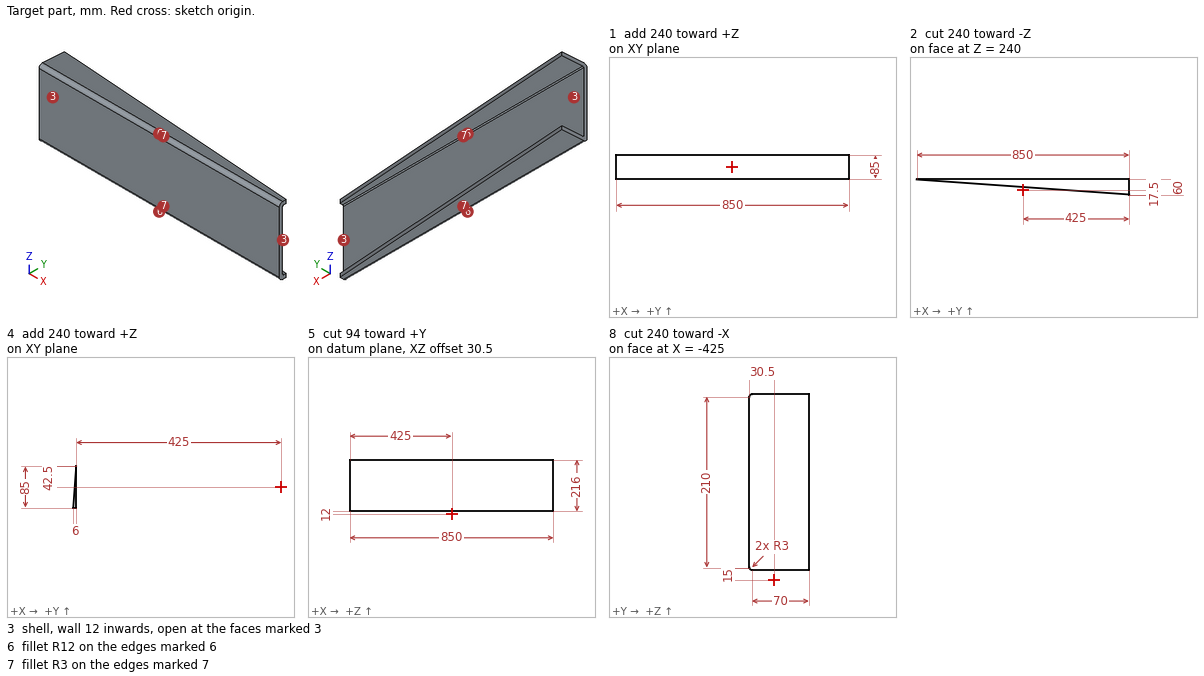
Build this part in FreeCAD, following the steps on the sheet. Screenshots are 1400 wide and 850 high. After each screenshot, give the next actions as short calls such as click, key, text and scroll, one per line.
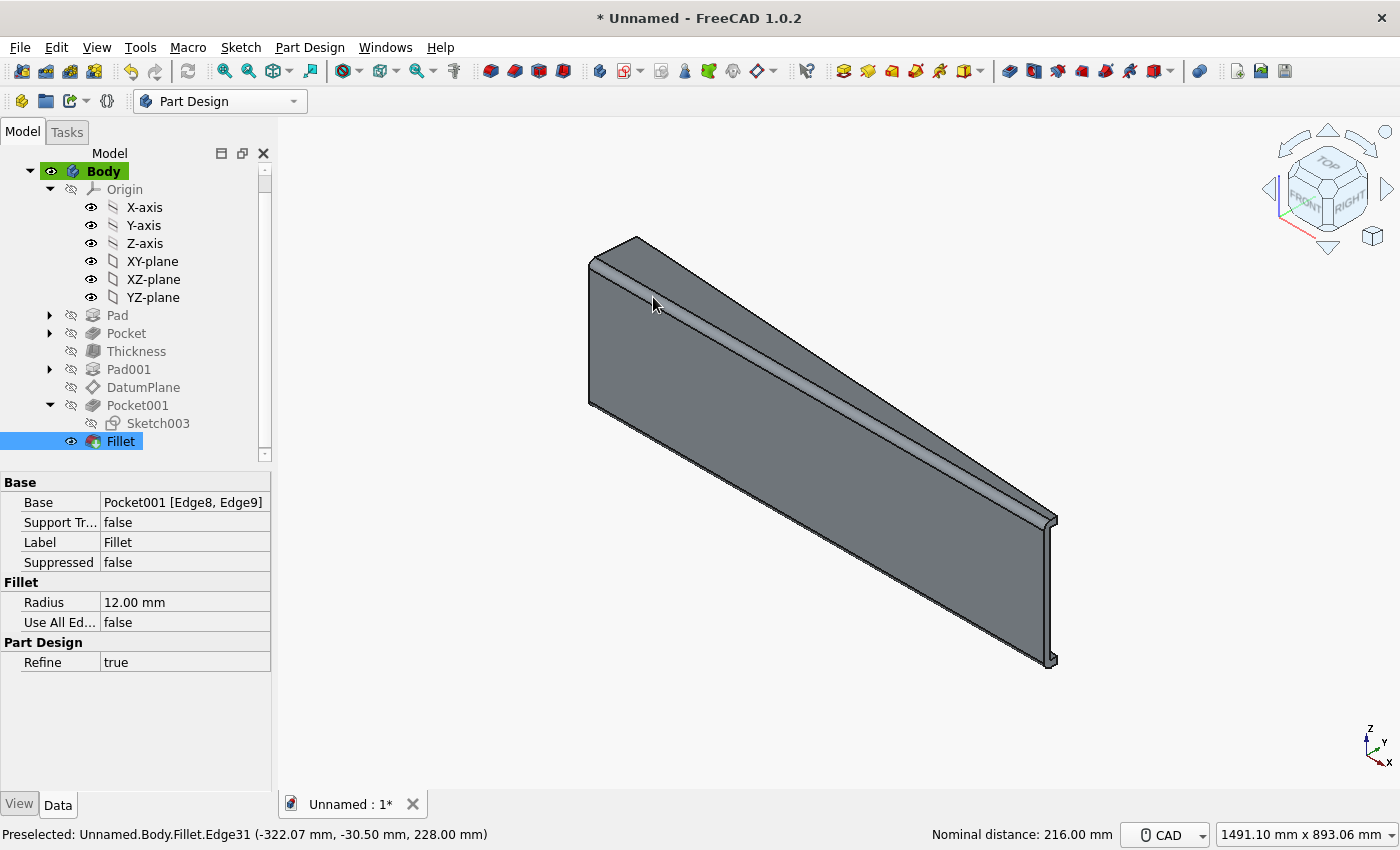
click(492, 72)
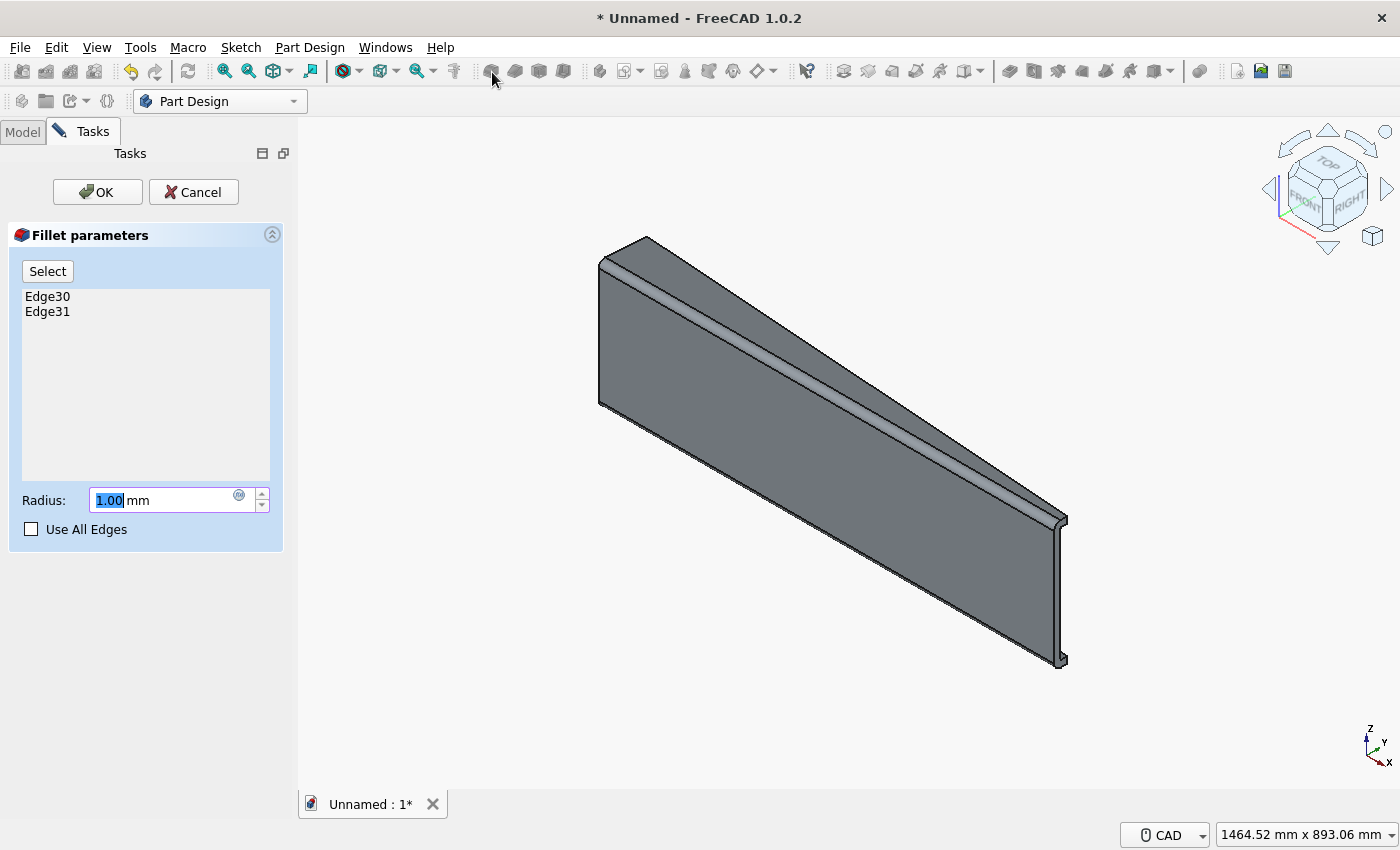
text(3)
key(Tab)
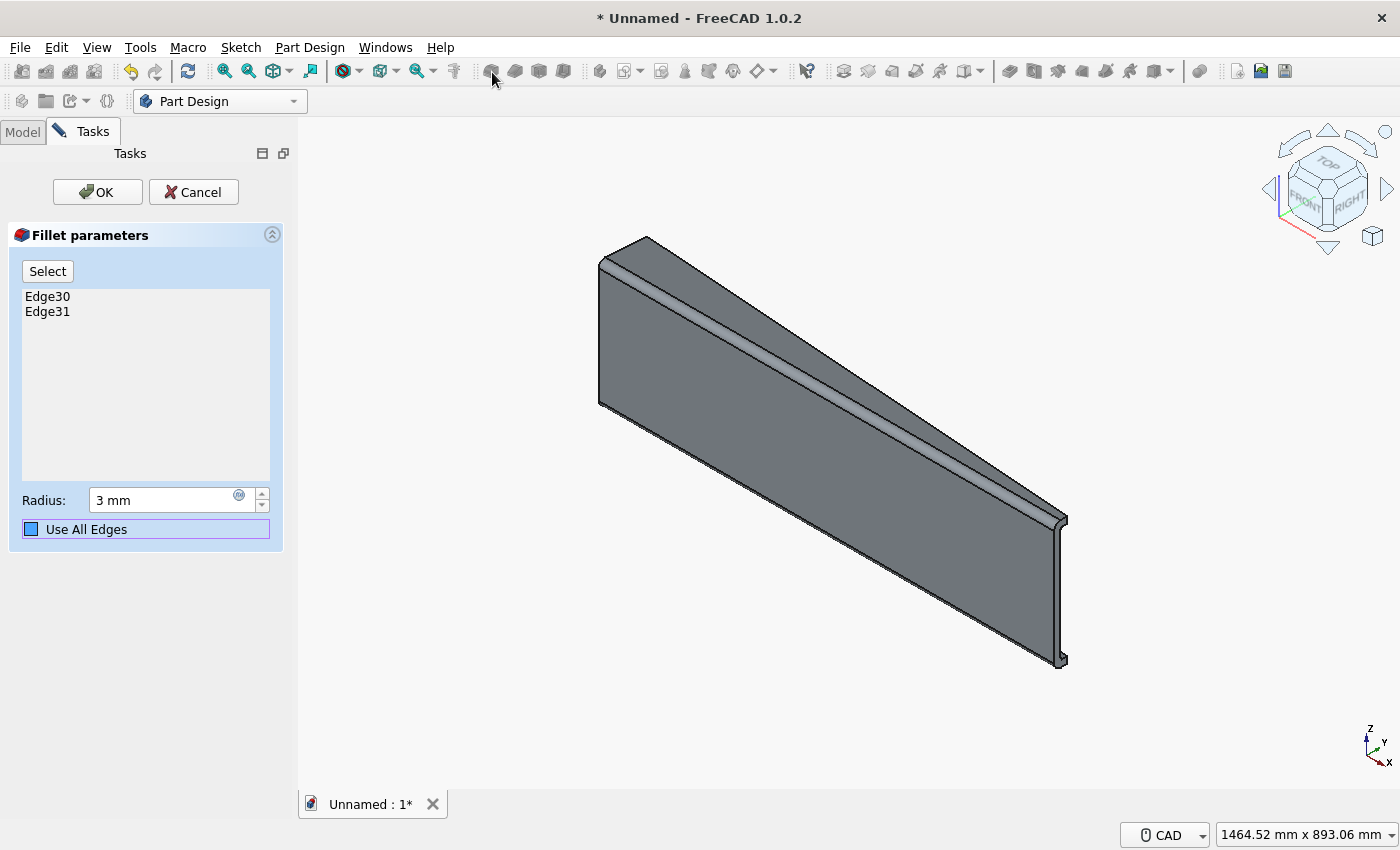
click(98, 192)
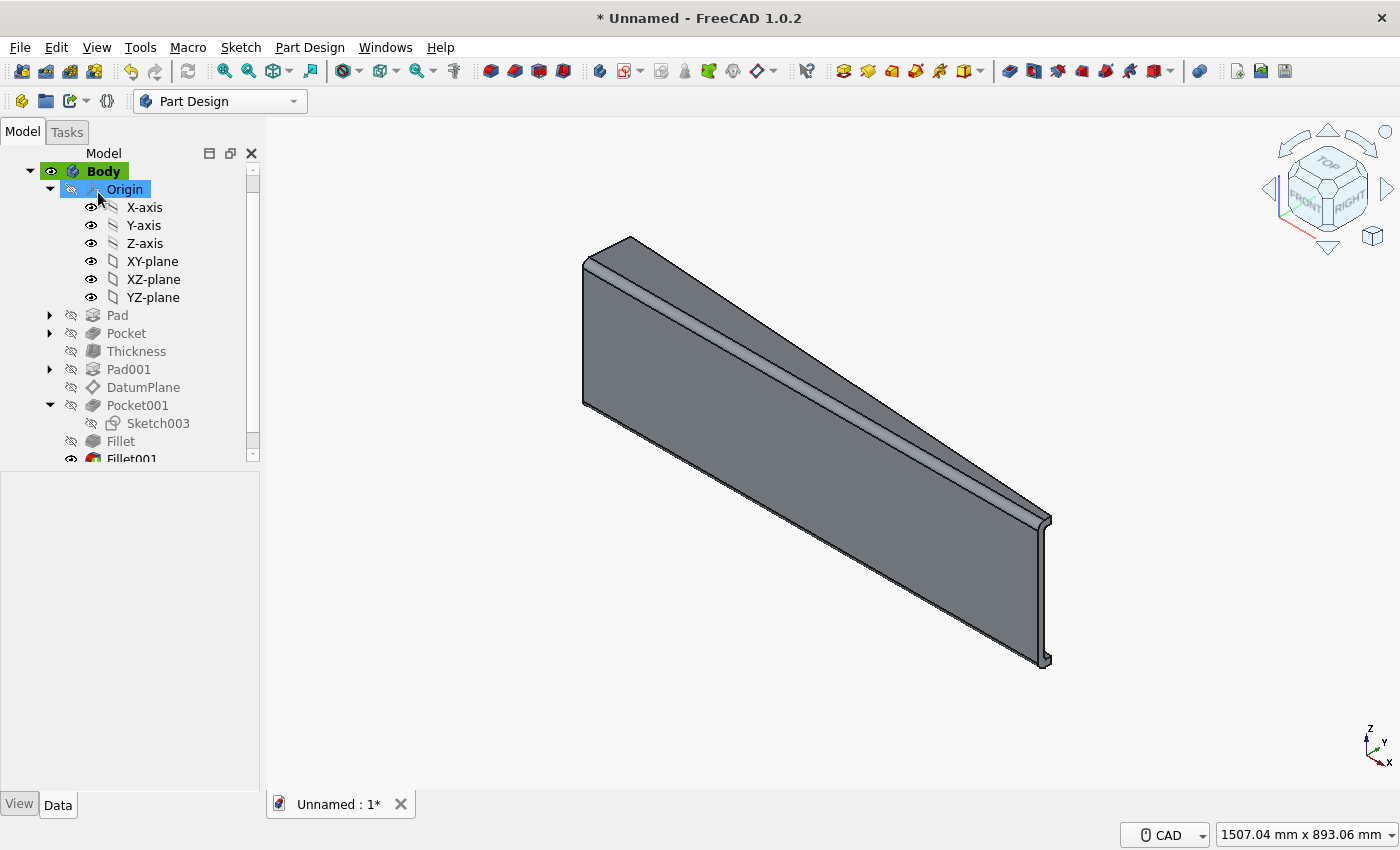
key(3)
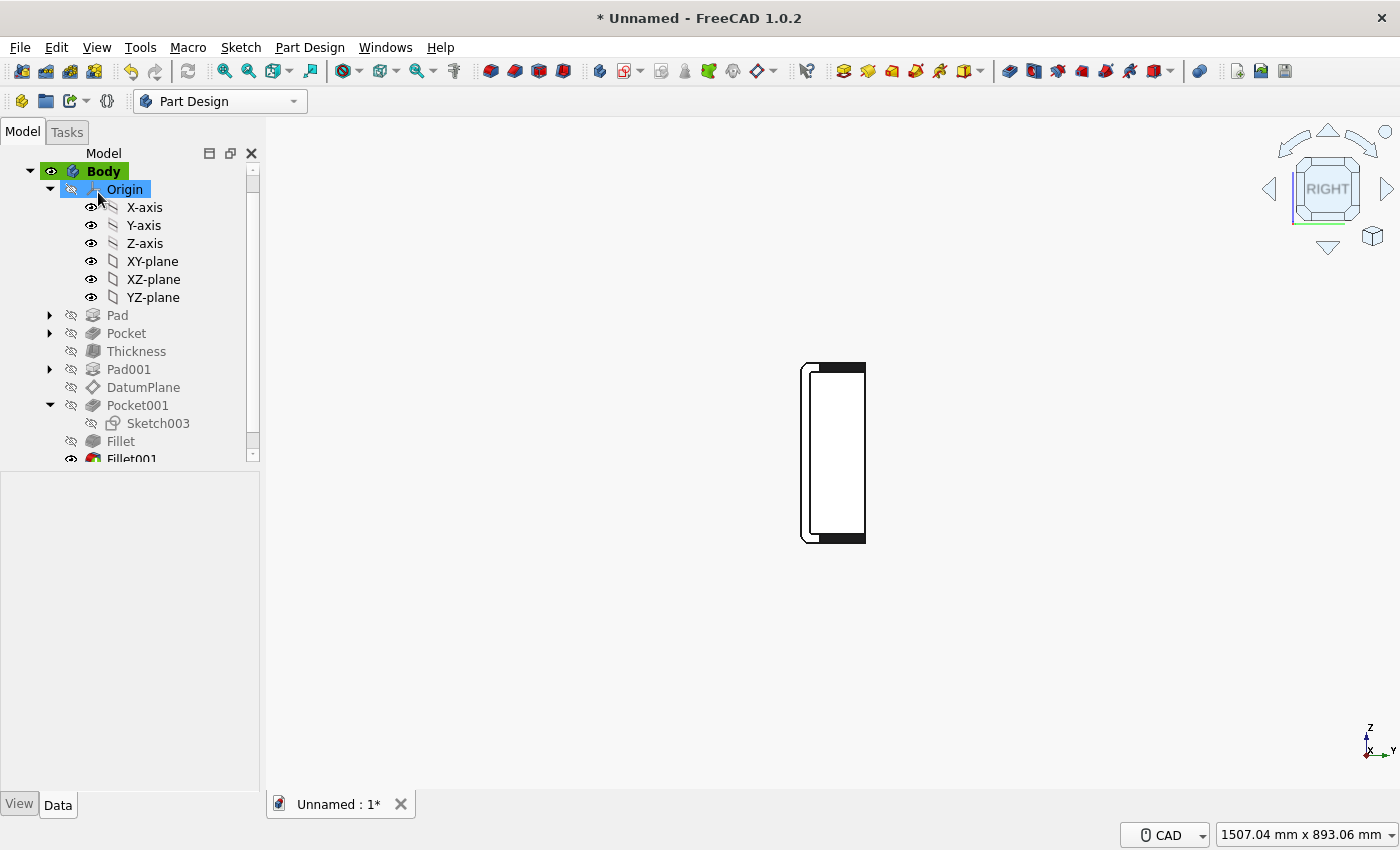
click(226, 72)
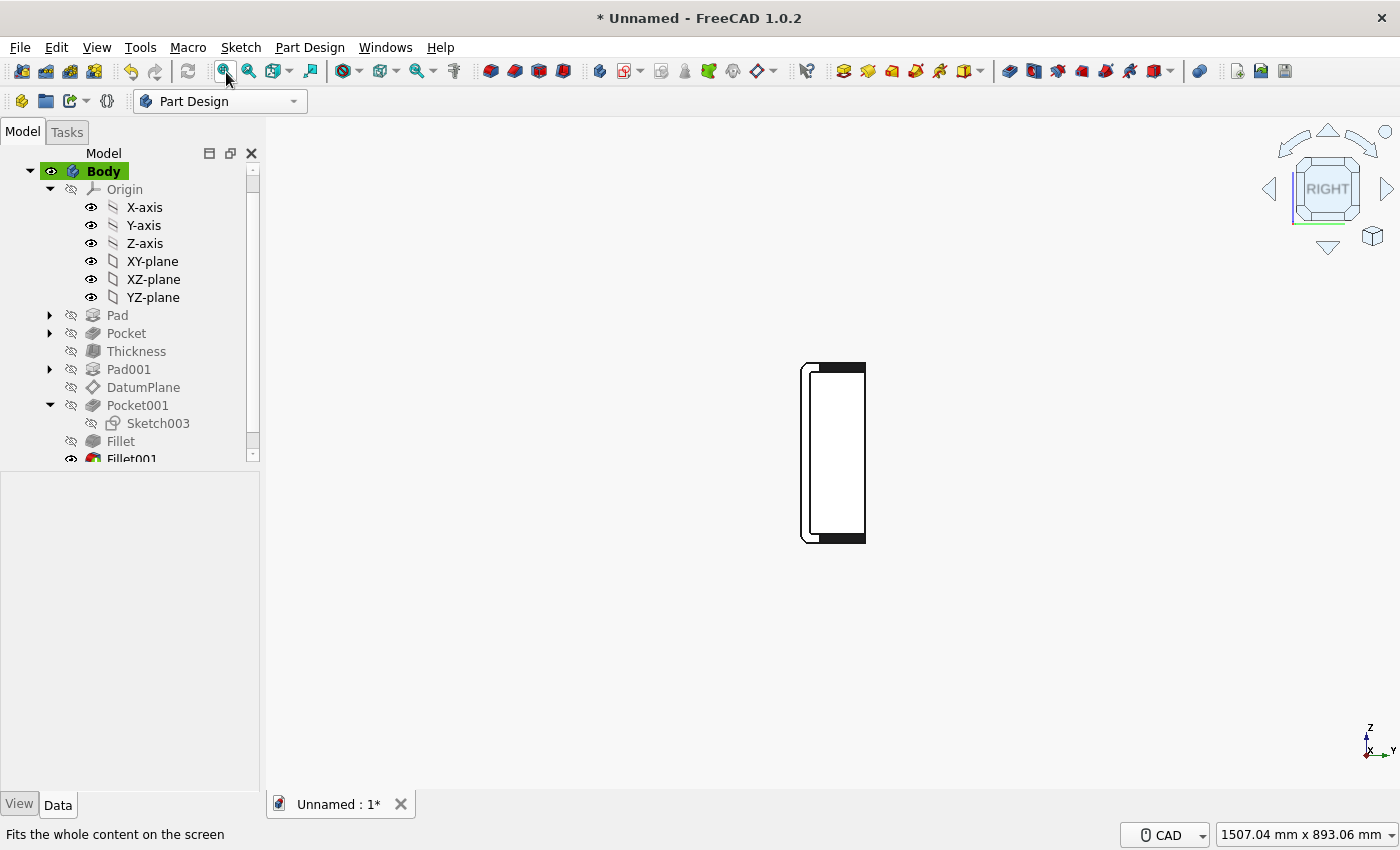
click(838, 406)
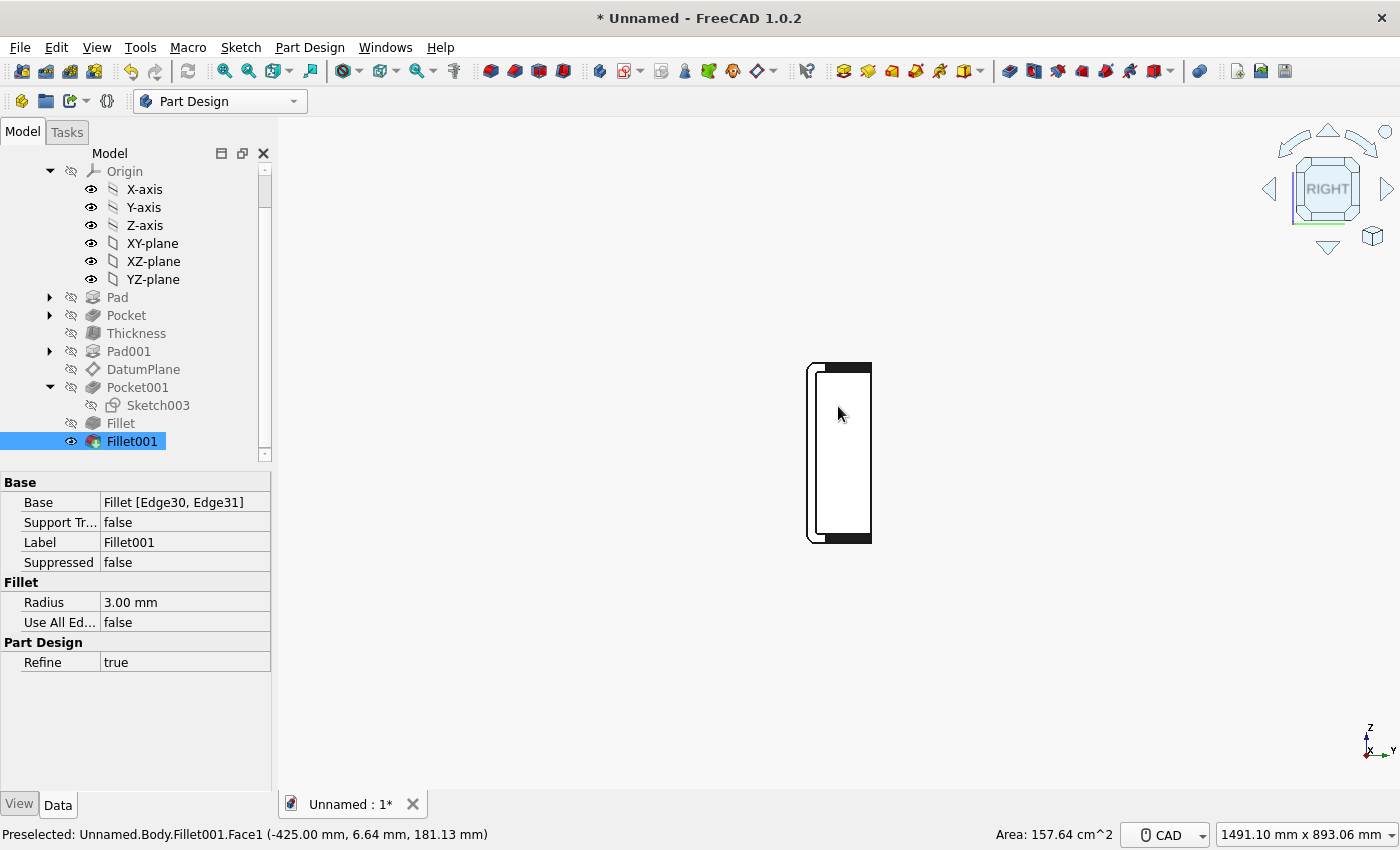
click(624, 72)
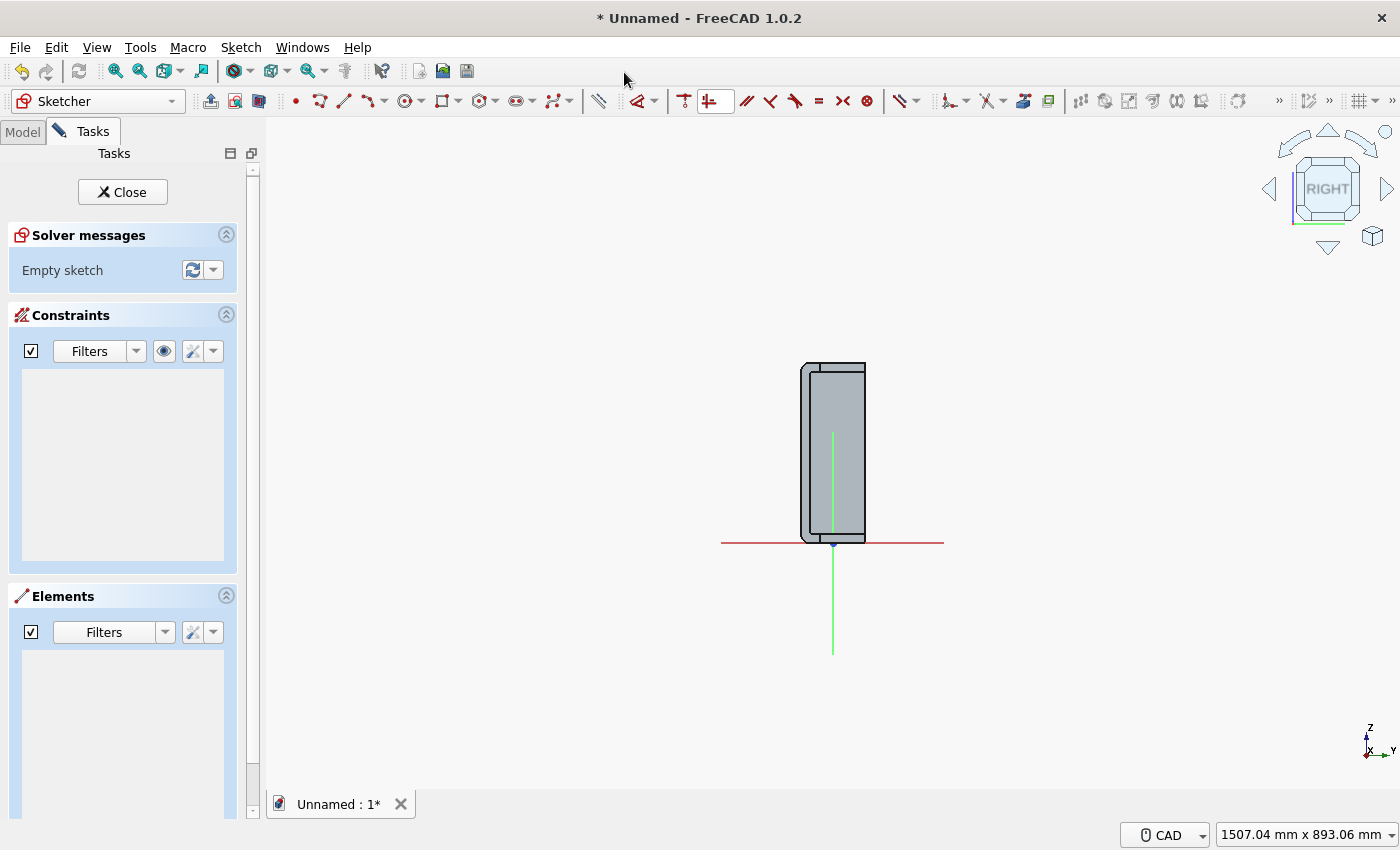
scroll(880, 460, up, 5)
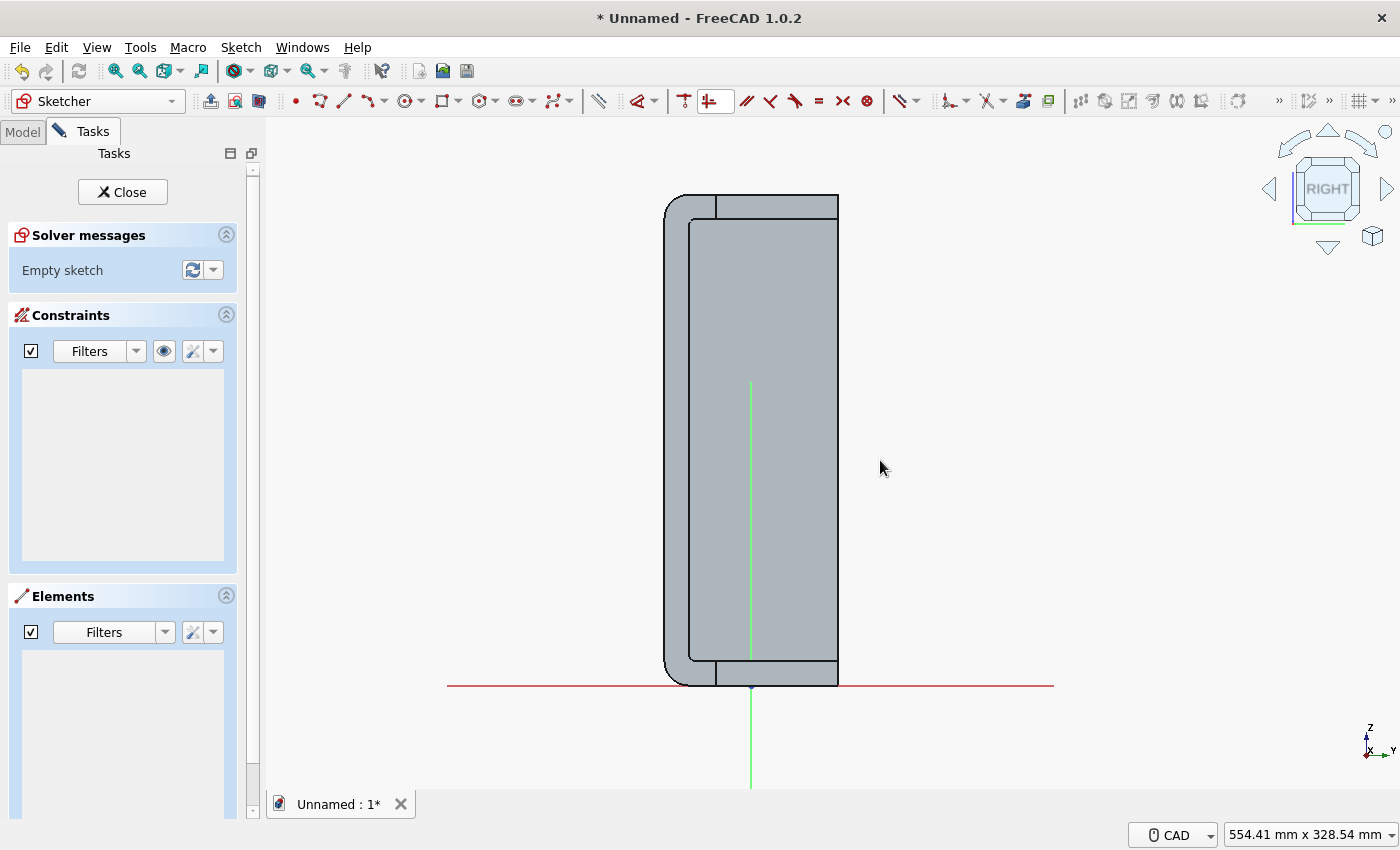
key(g)
key(l)